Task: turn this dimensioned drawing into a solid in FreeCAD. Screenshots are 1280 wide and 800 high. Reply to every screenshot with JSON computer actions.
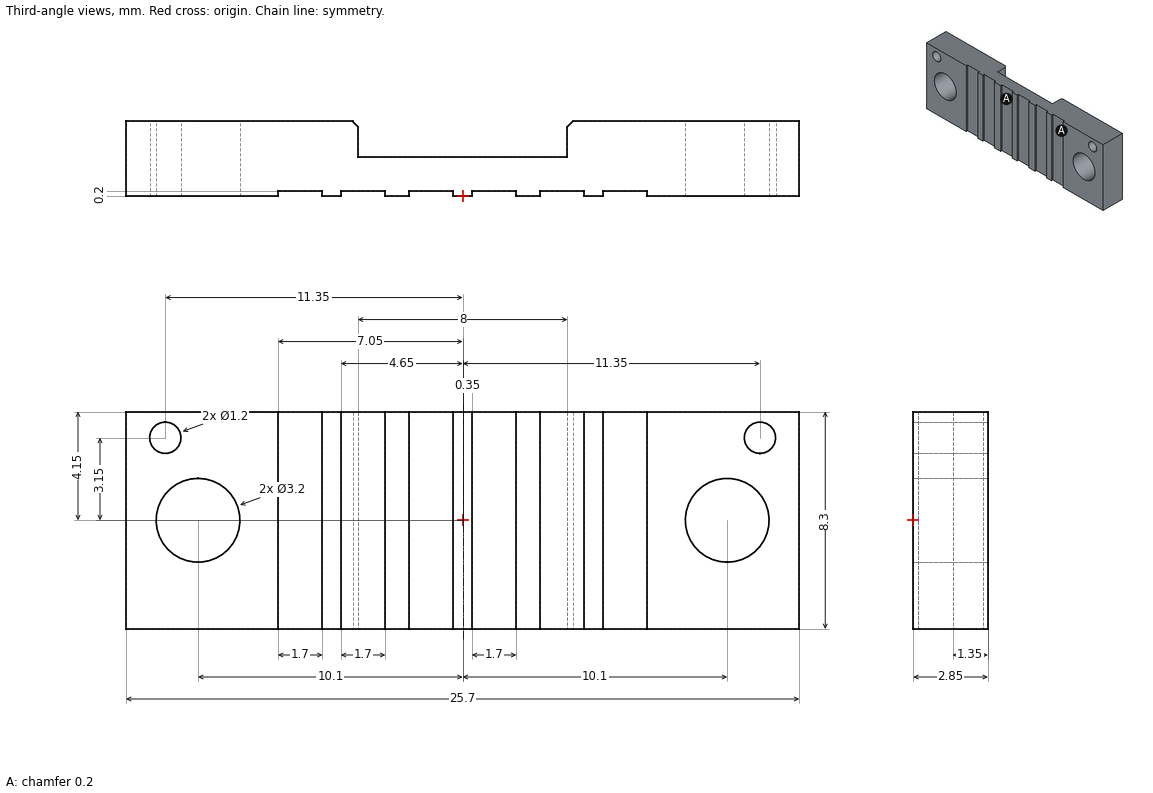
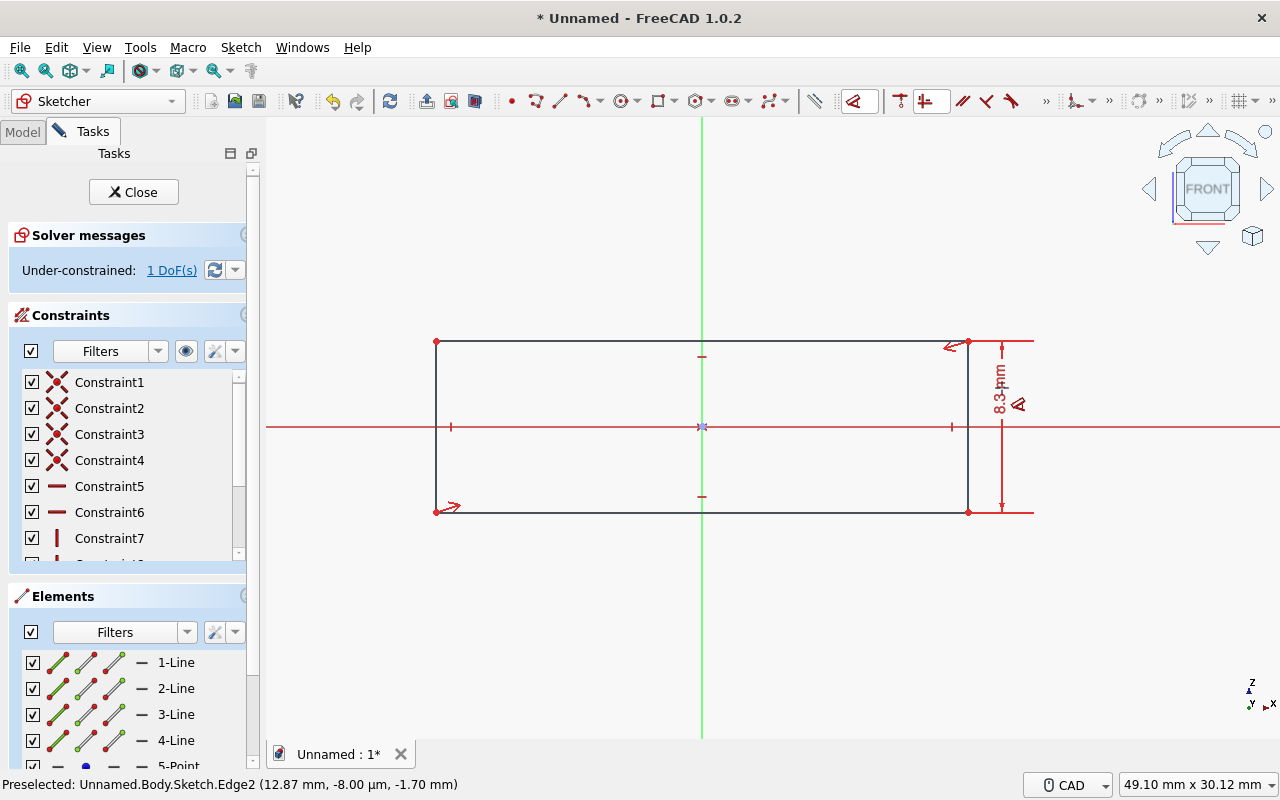
{"action": "left_click", "coordinate": [596, 513]}
{"action": "left_click", "coordinate": [580, 547]}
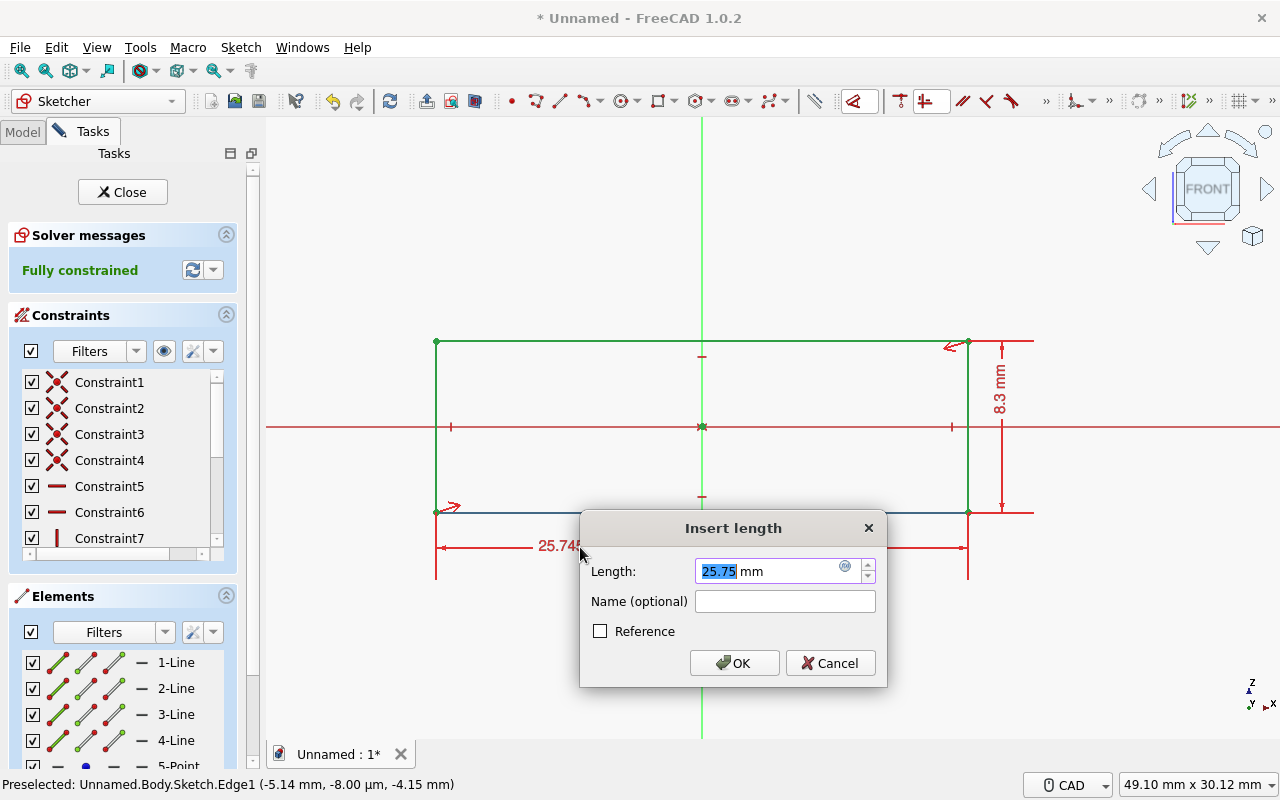
{"action": "type", "text": "25.7"}
{"action": "key", "text": "Return"}
{"action": "key", "text": "Escape"}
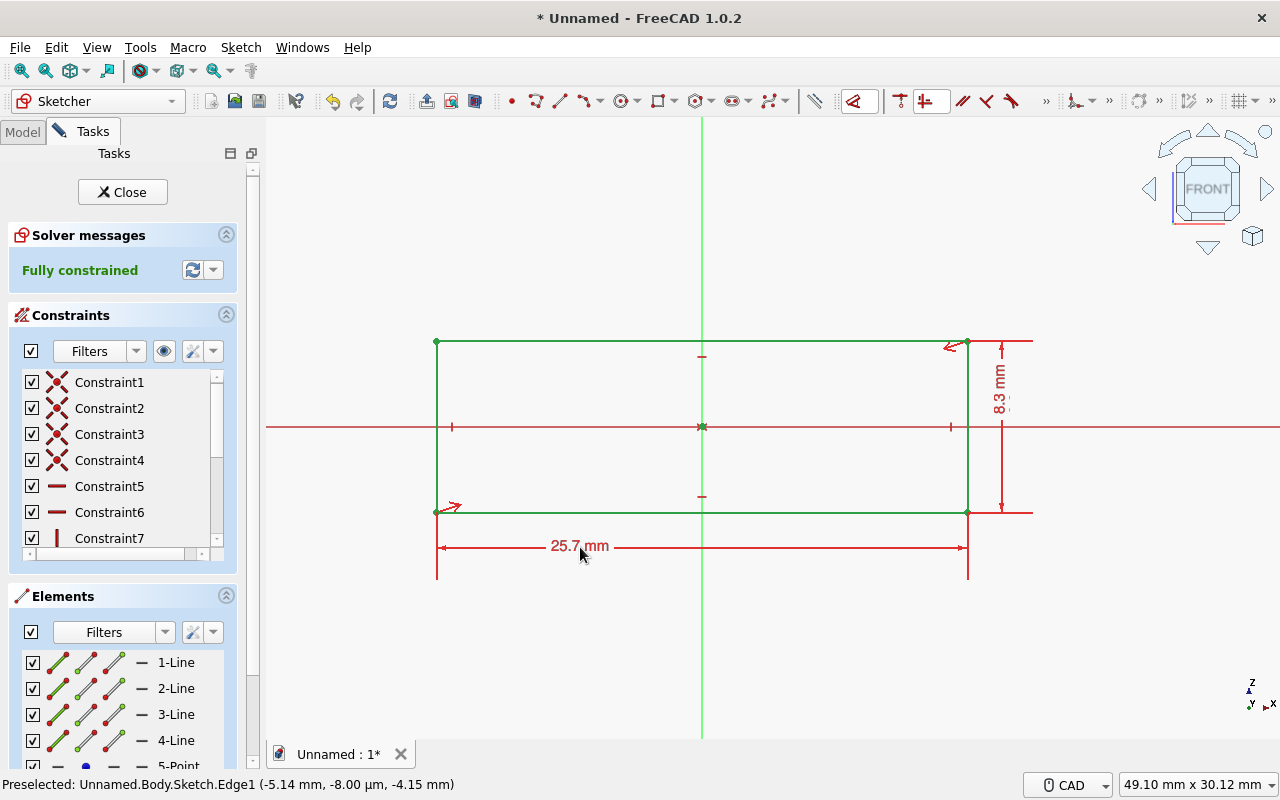
{"action": "left_click", "coordinate": [123, 192]}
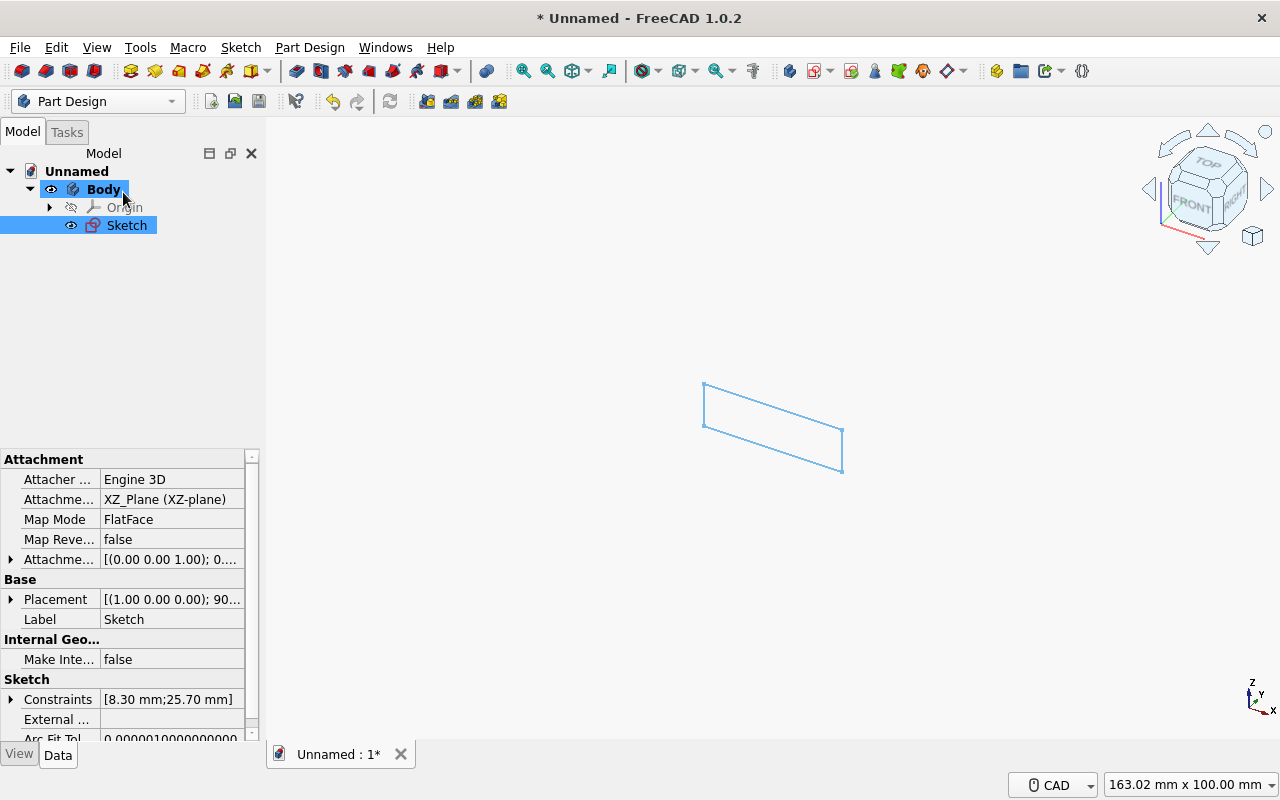
{"action": "left_click", "coordinate": [132, 72]}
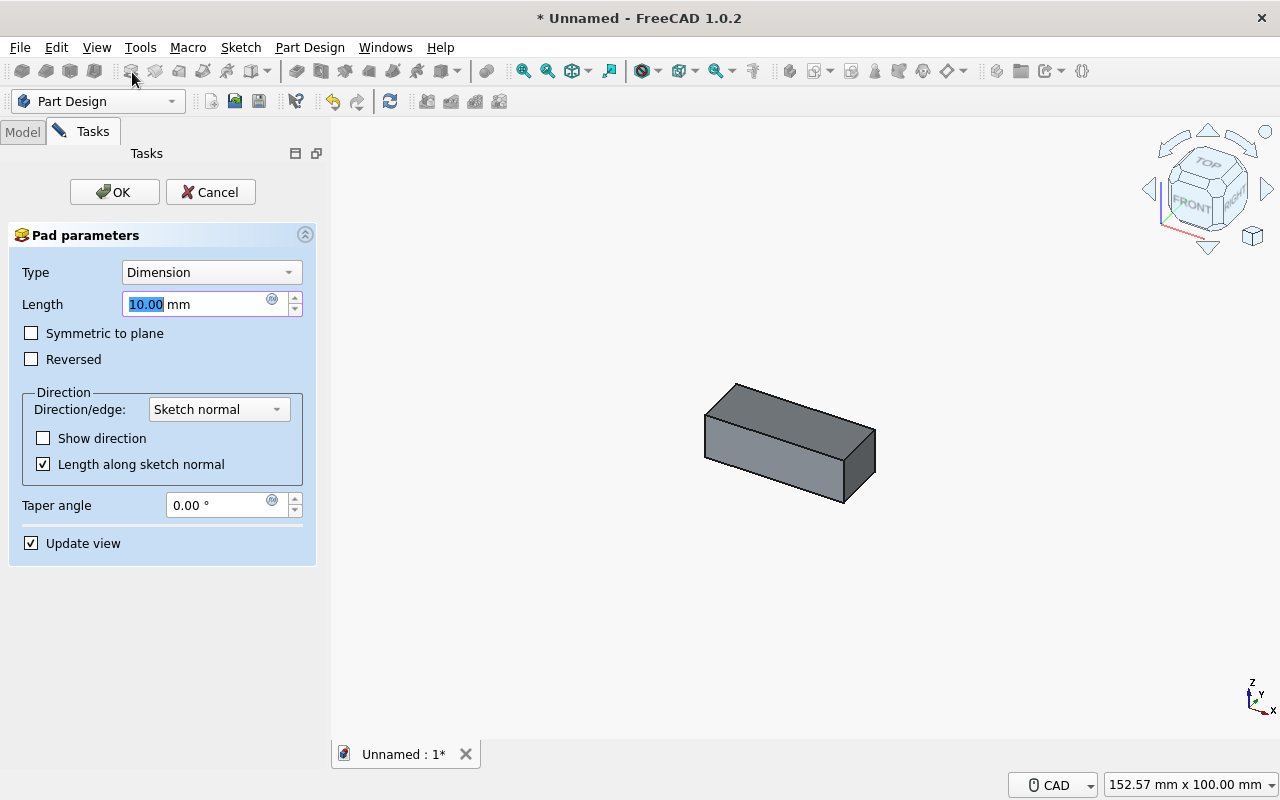
{"action": "type", "text": "2.85"}
{"action": "key", "text": "Tab"}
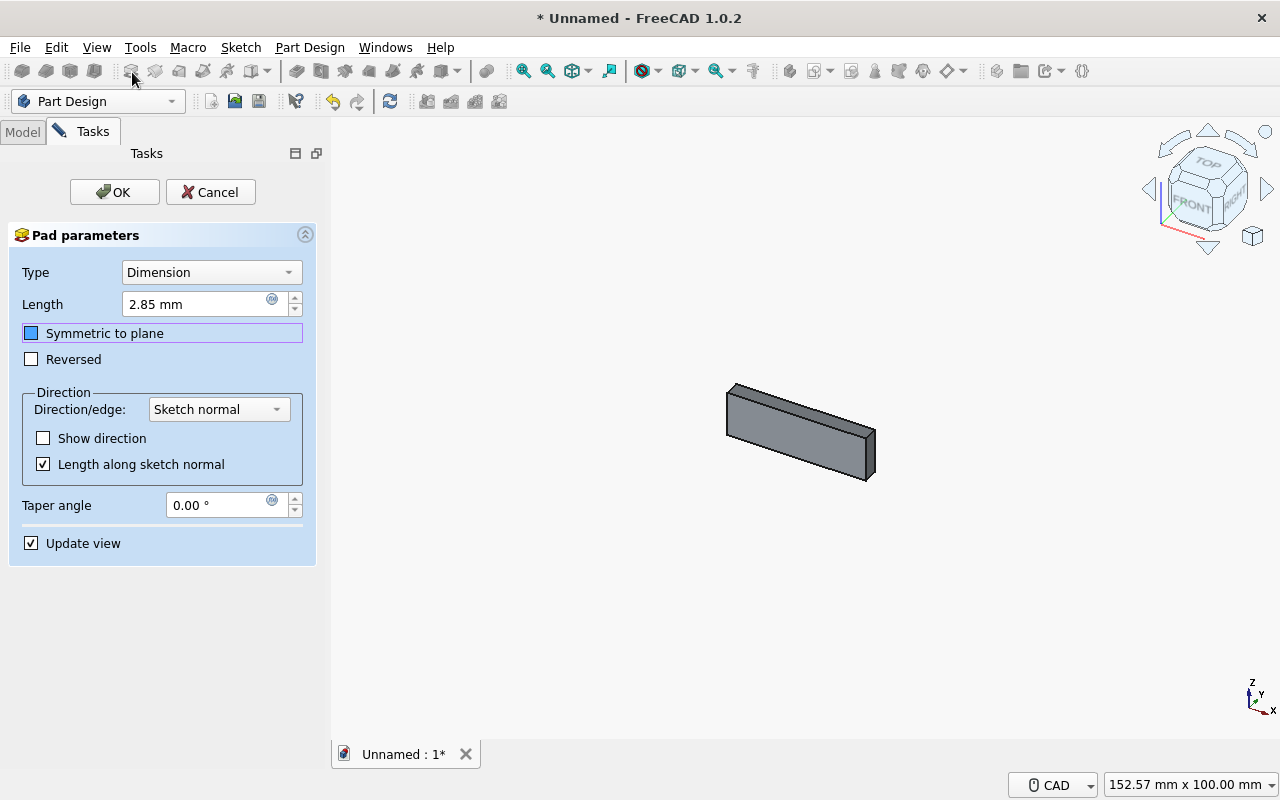
{"action": "left_click", "coordinate": [30, 359]}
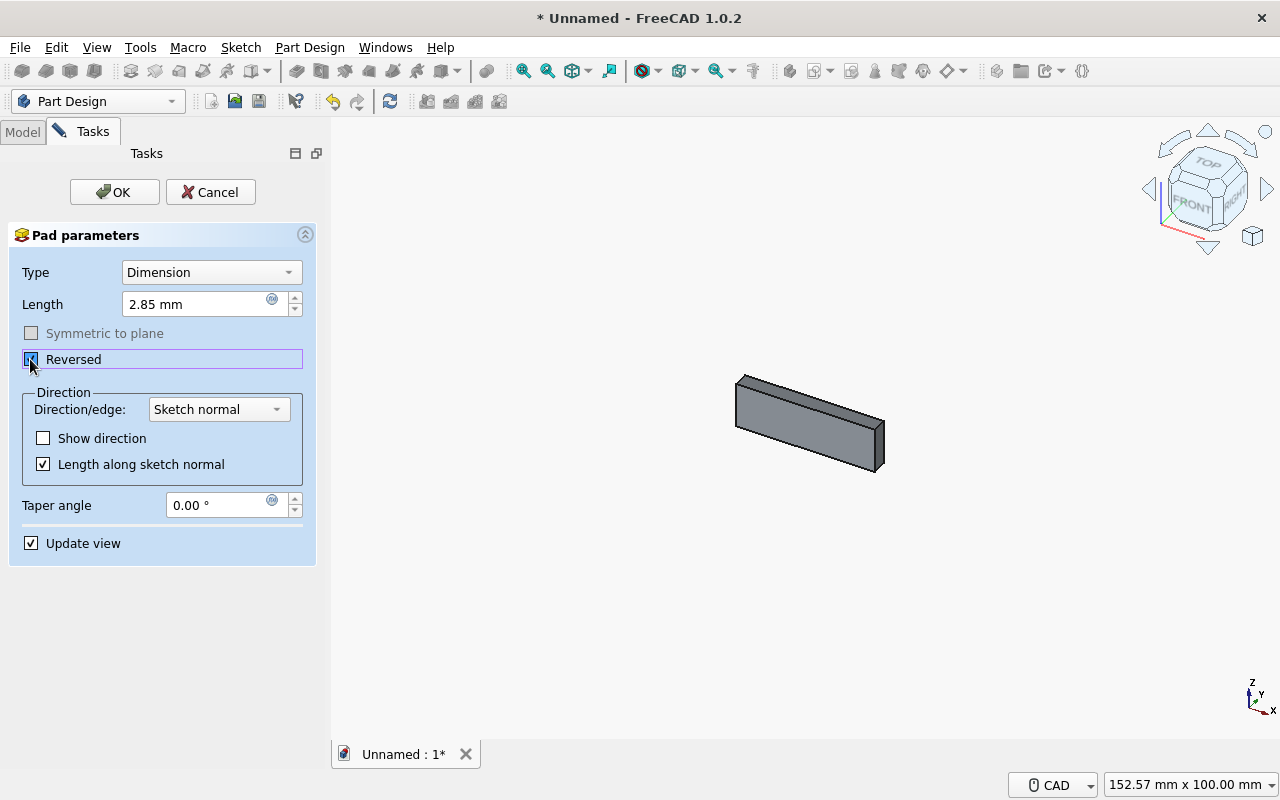
{"action": "left_click", "coordinate": [115, 192]}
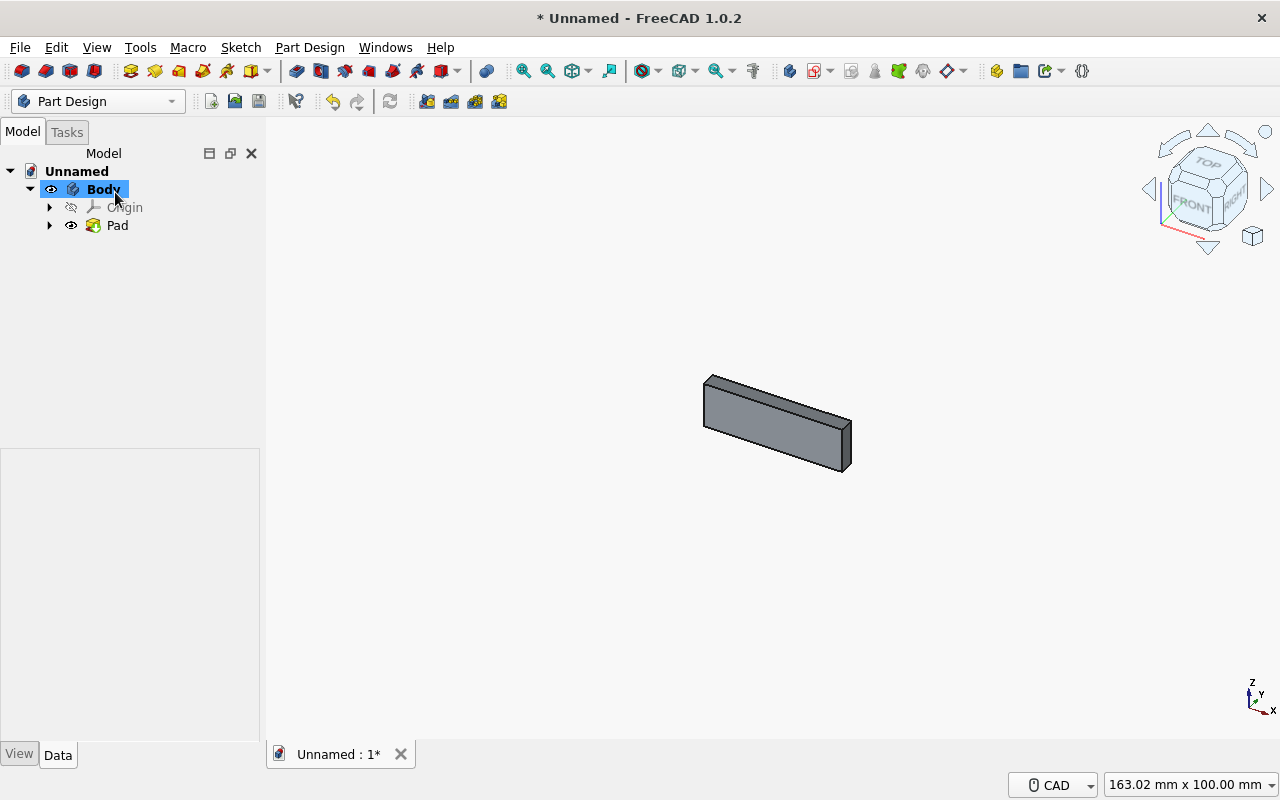
{"action": "key", "text": "v f"}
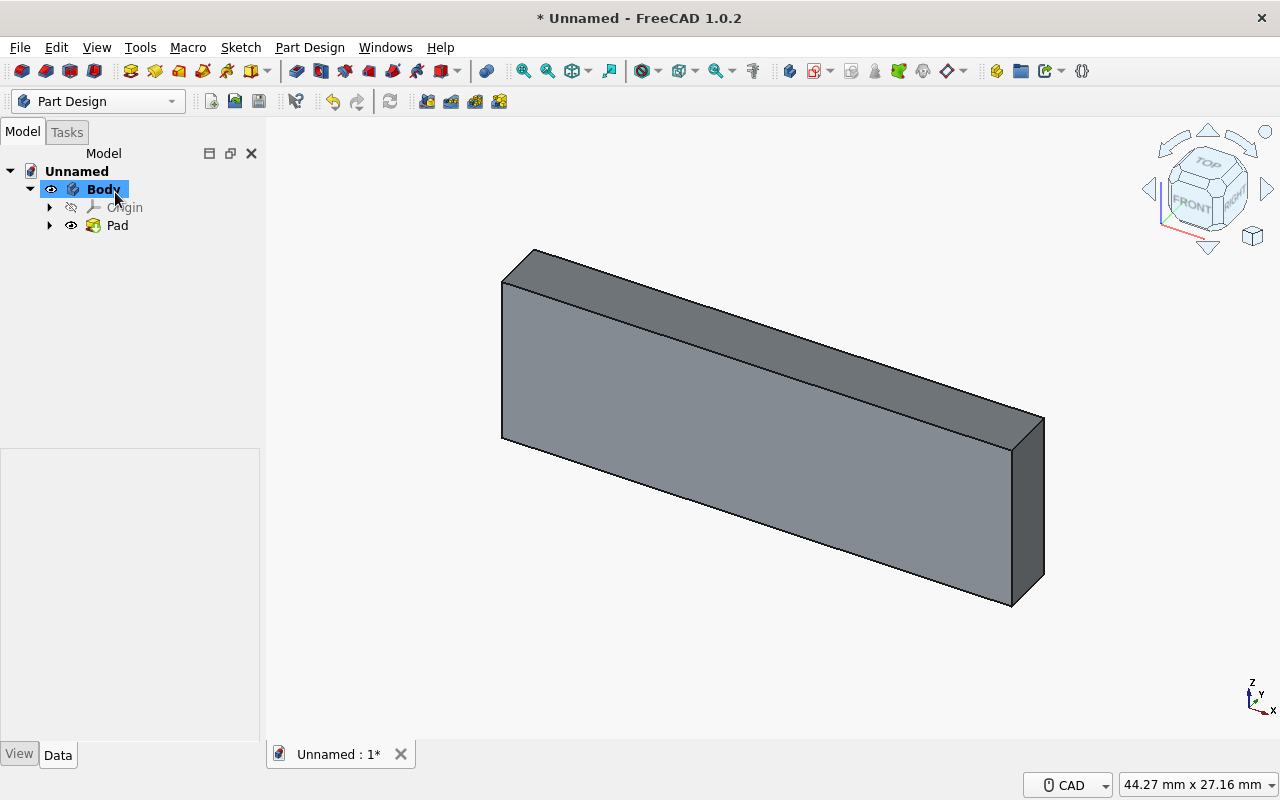
{"action": "key", "text": "4"}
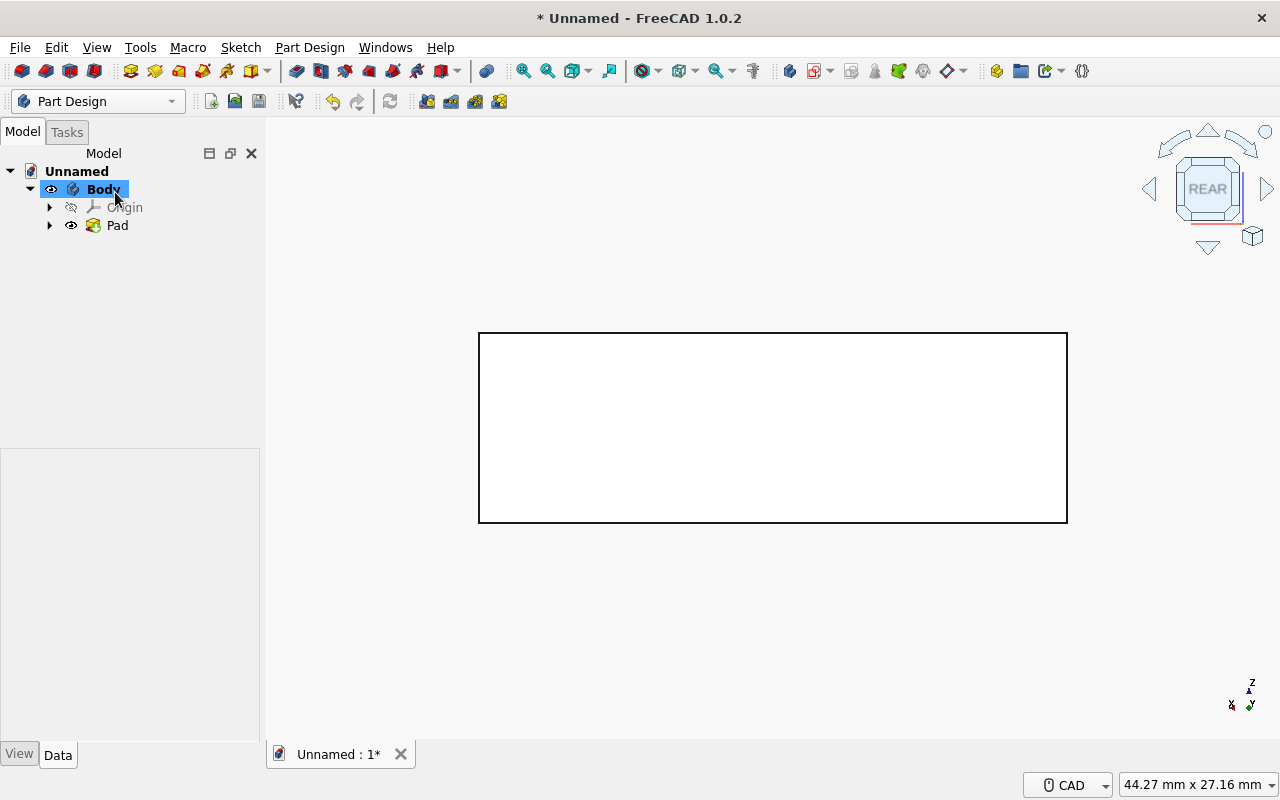
{"action": "left_click", "coordinate": [605, 427]}